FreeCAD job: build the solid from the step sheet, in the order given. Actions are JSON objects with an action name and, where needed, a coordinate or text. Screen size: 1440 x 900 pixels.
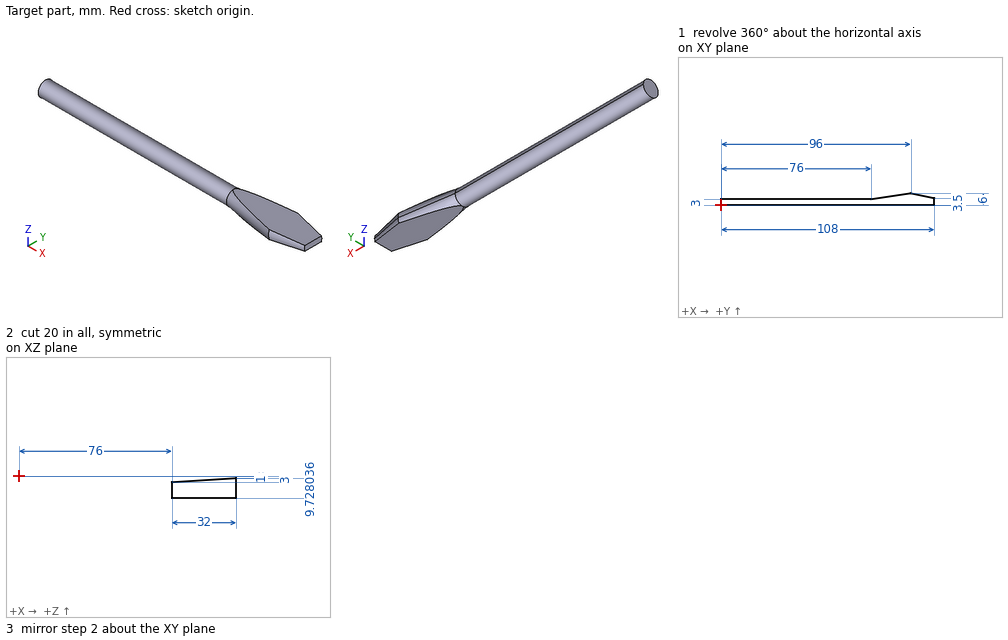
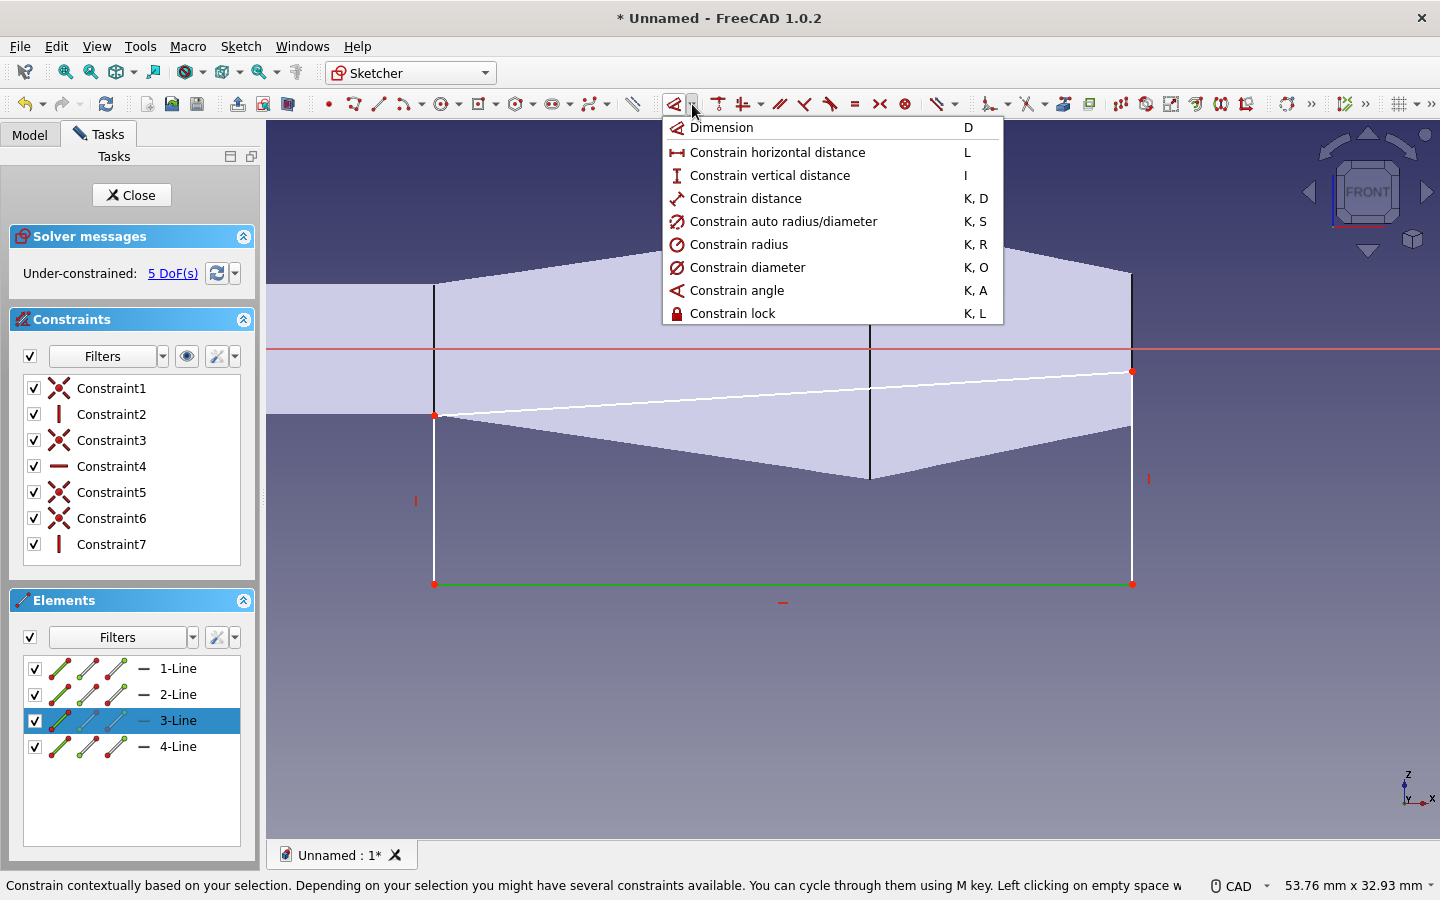
{"action": "left_click", "coordinate": [833, 152]}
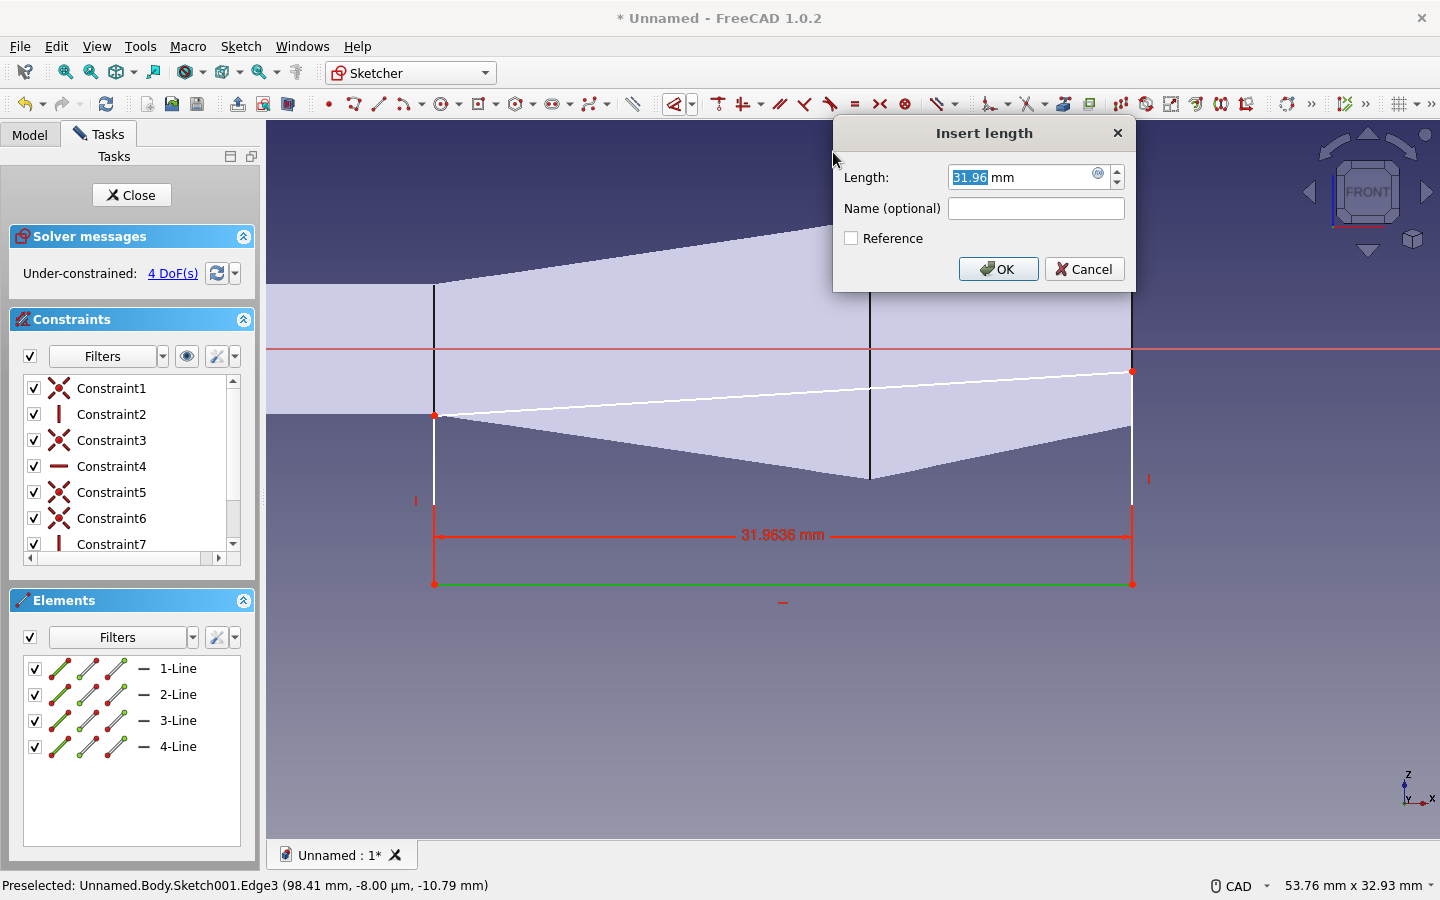
{"action": "type", "text": "32"}
{"action": "key", "text": "Return"}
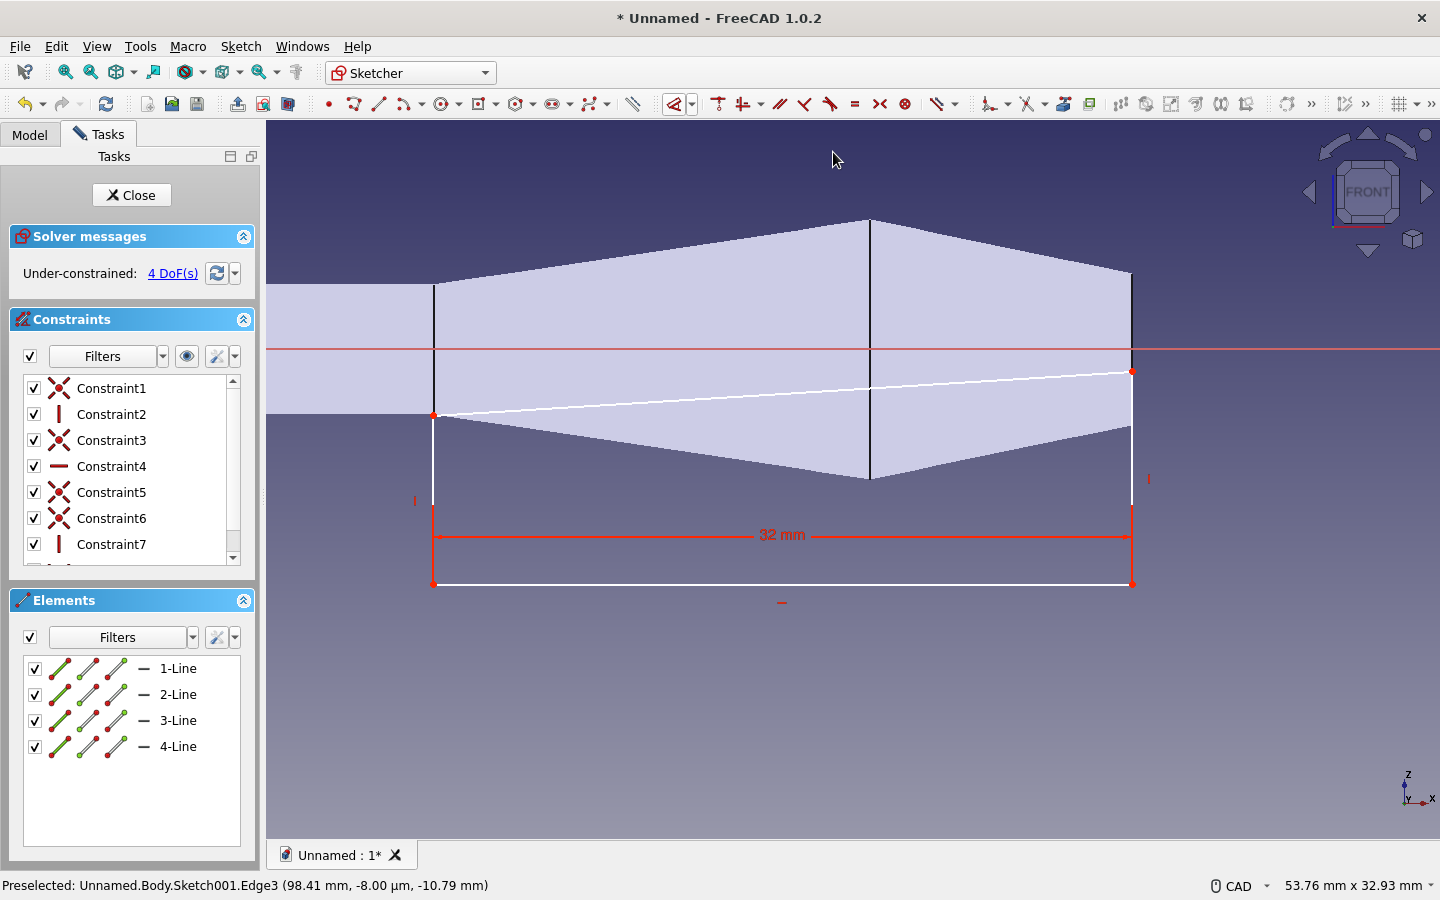
{"action": "left_click", "coordinate": [433, 416]}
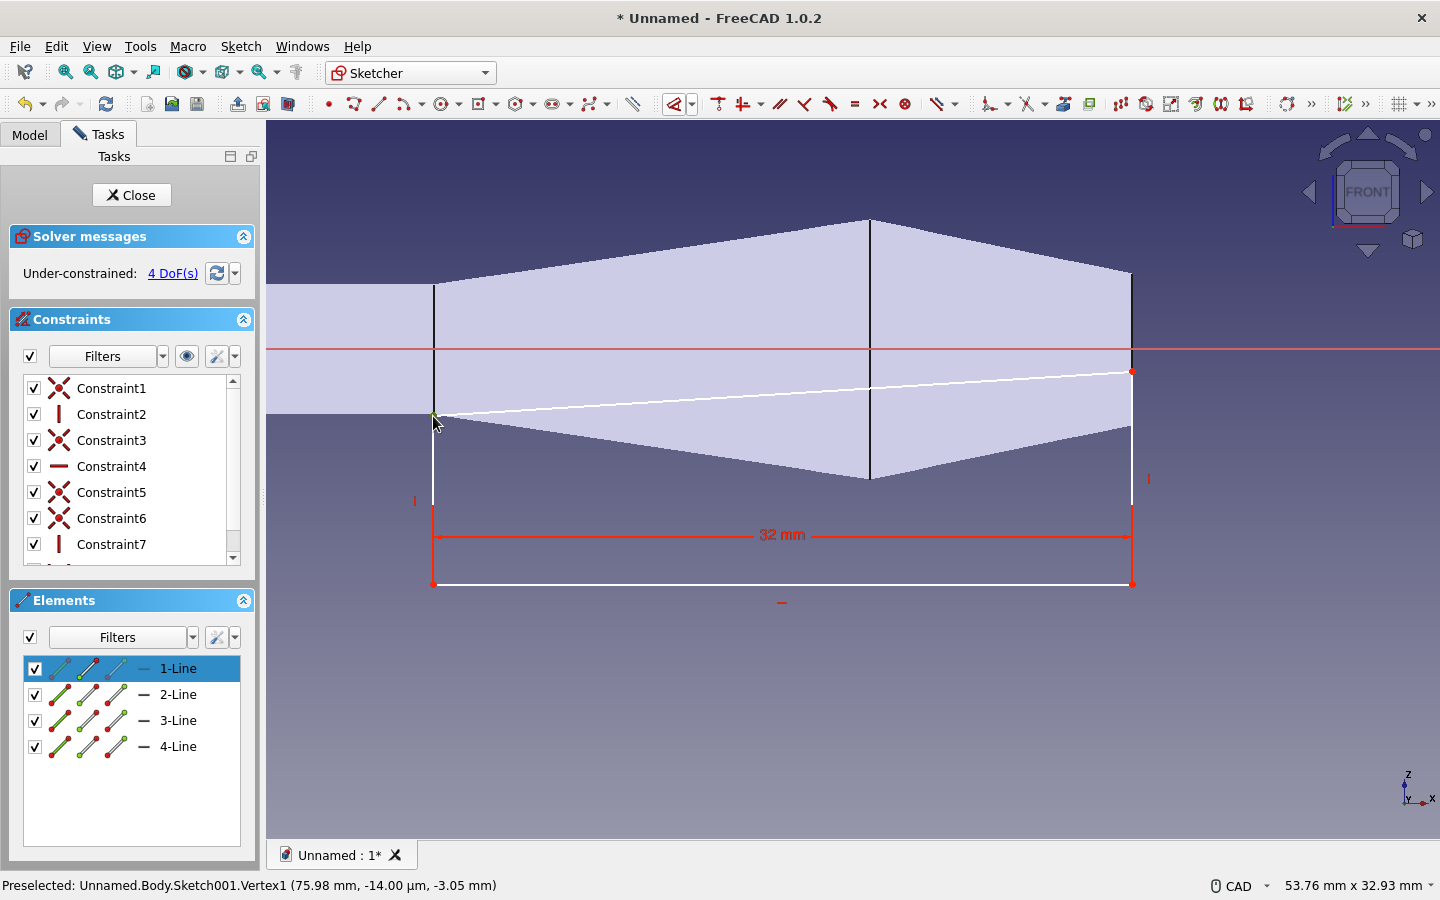
{"action": "key", "text": "i"}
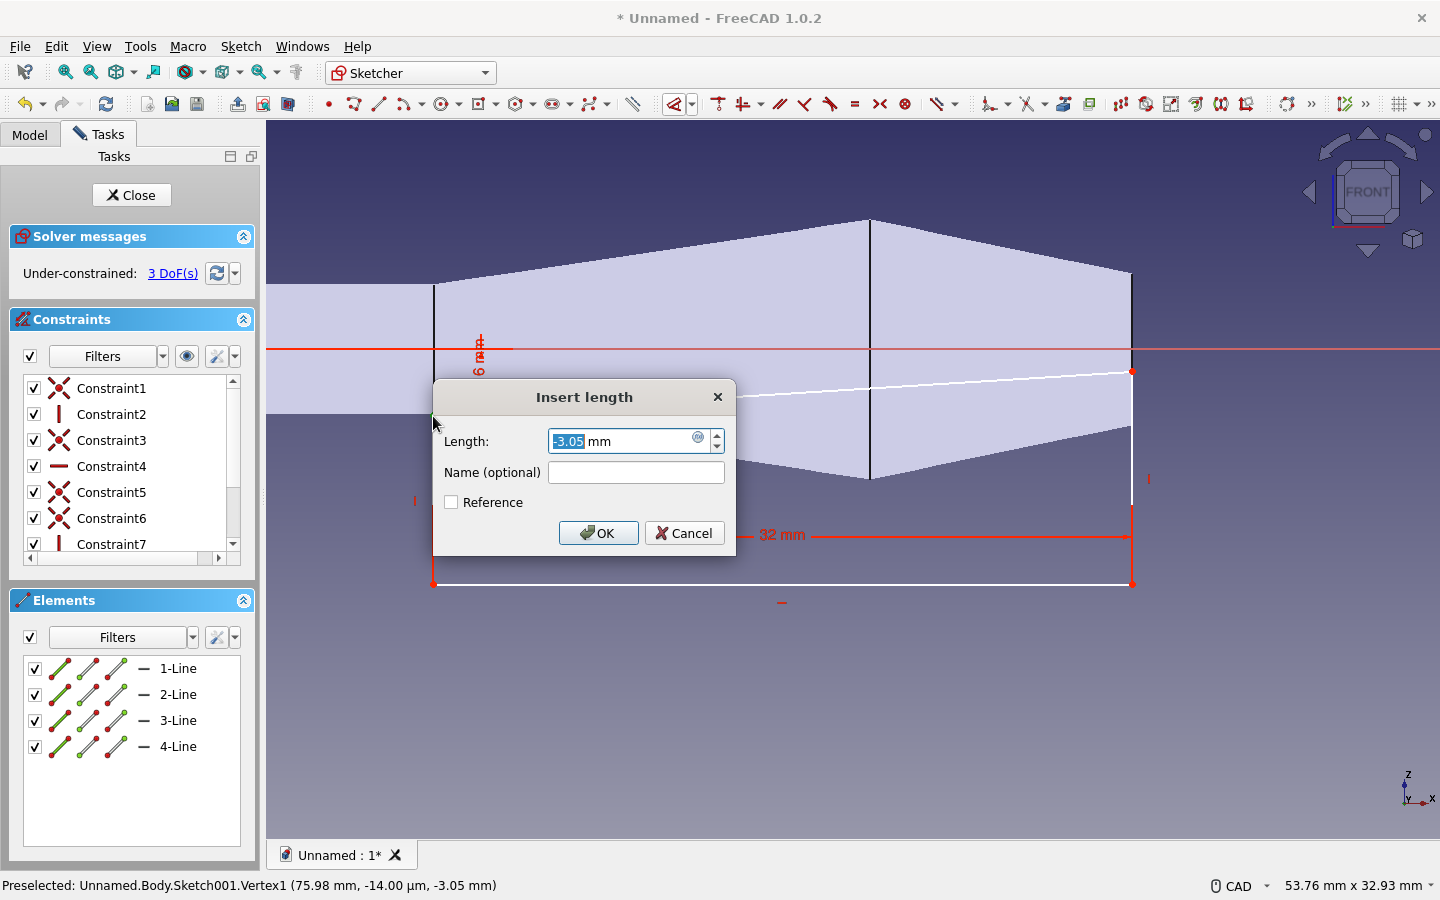
{"action": "type", "text": "-3"}
{"action": "key", "text": "Return"}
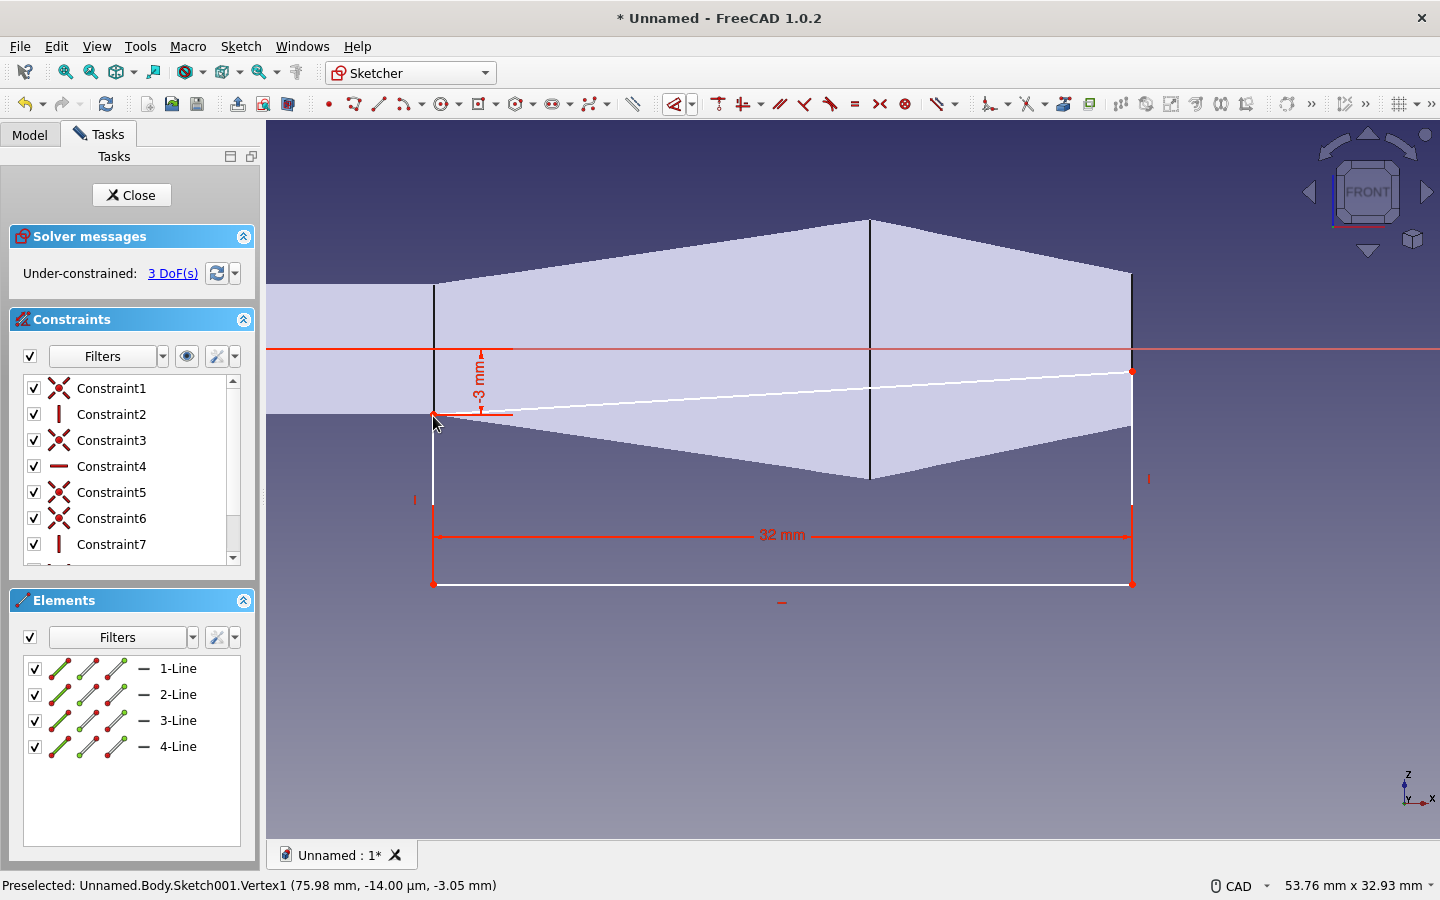
{"action": "scroll", "coordinate": [1132, 372], "scroll_direction": "up", "scroll_amount": 3}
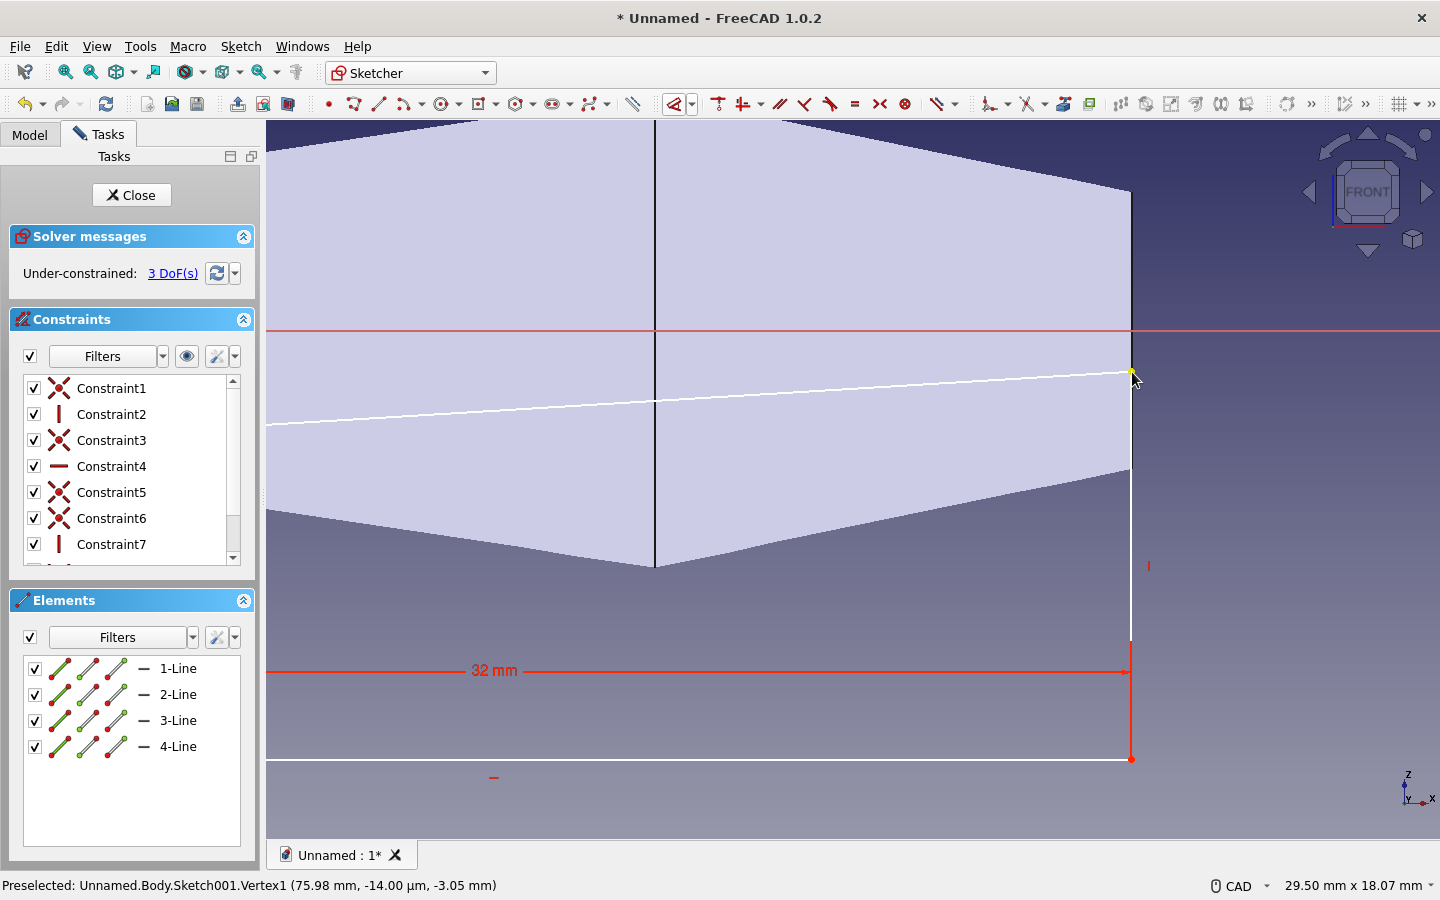
{"action": "left_click", "coordinate": [1131, 372]}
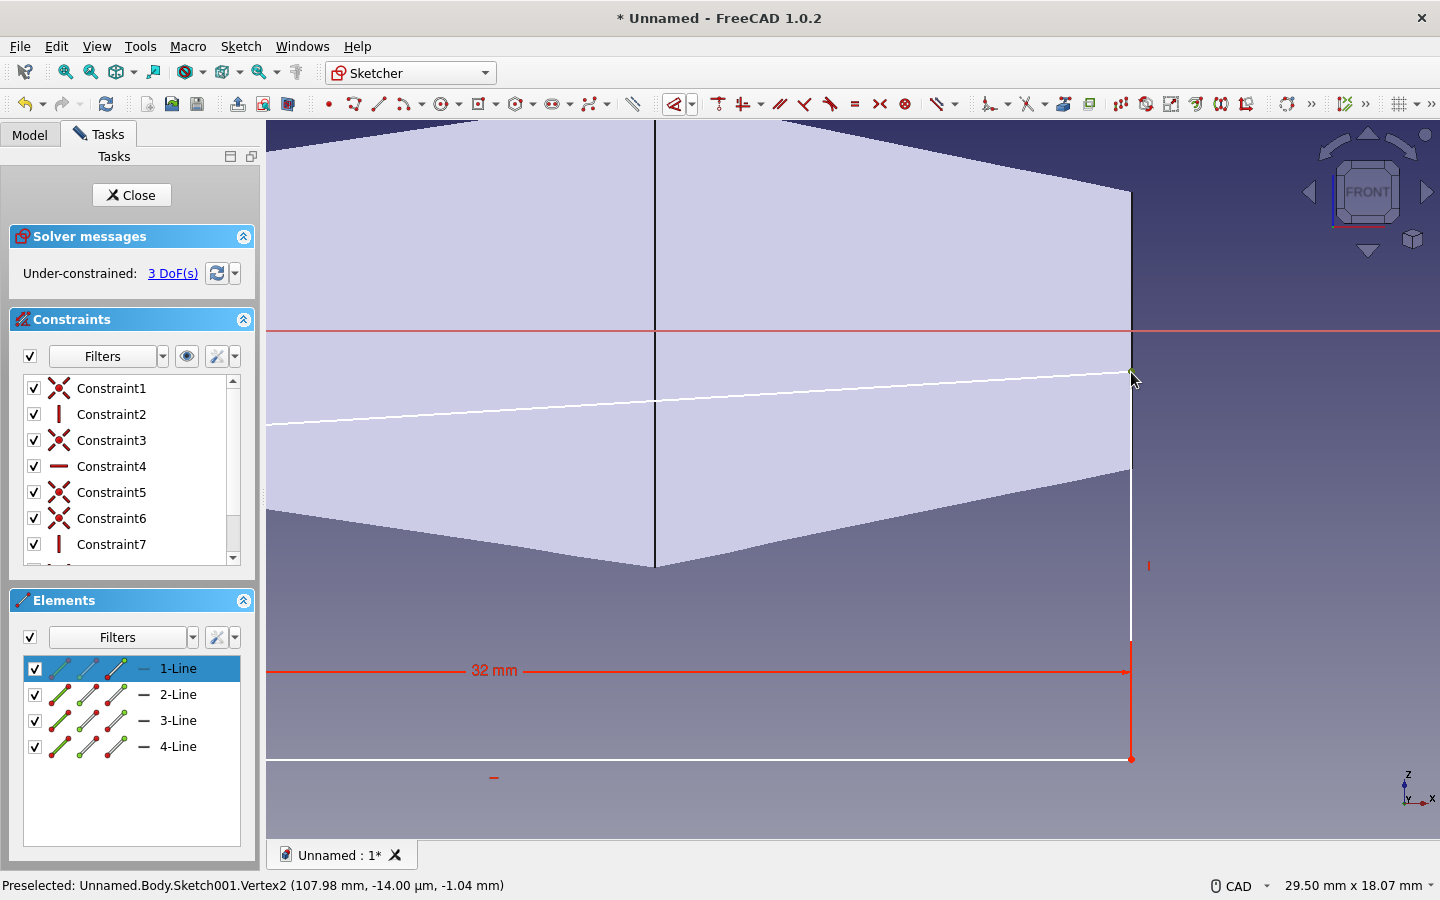
{"action": "key", "text": "i"}